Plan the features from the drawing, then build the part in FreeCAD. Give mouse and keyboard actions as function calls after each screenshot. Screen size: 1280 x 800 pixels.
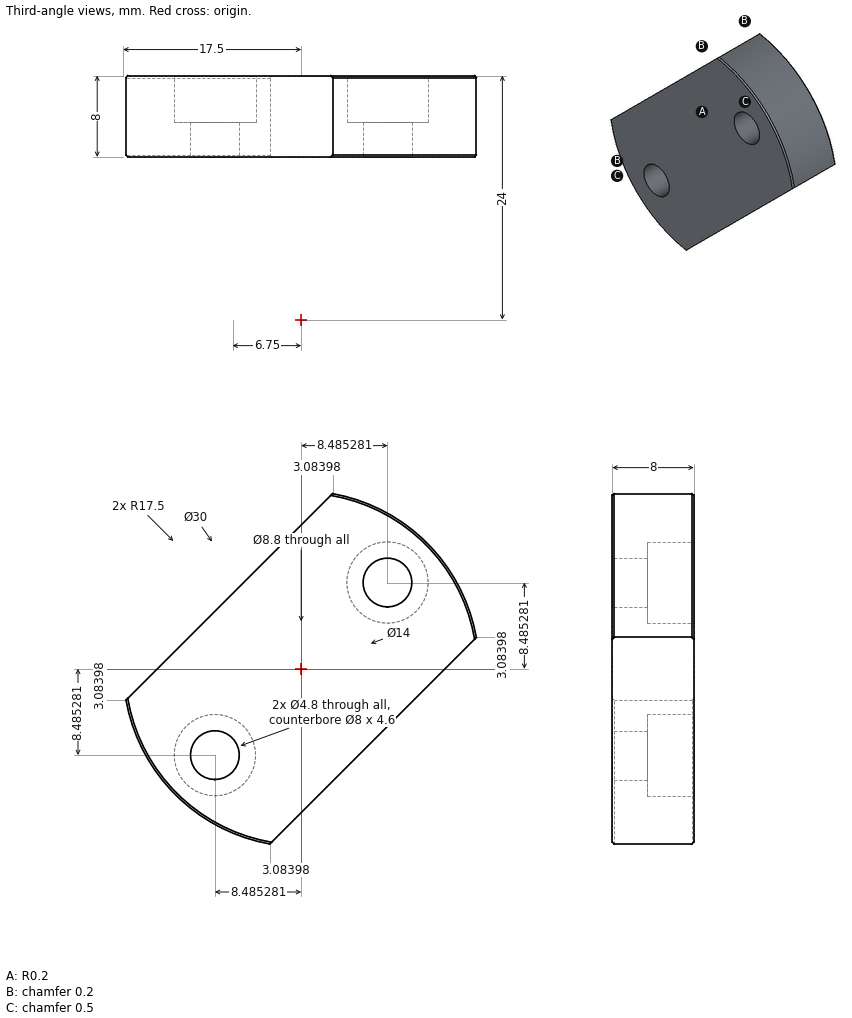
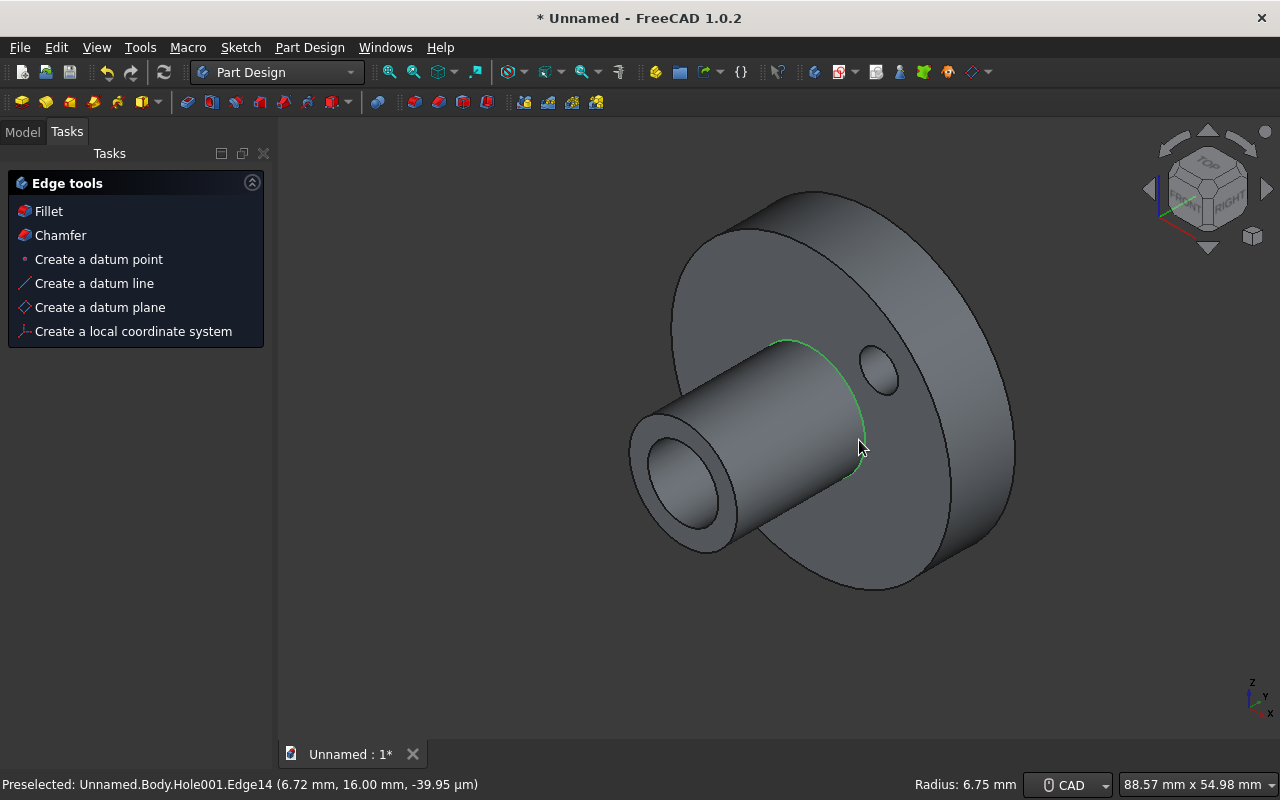
click(416, 102)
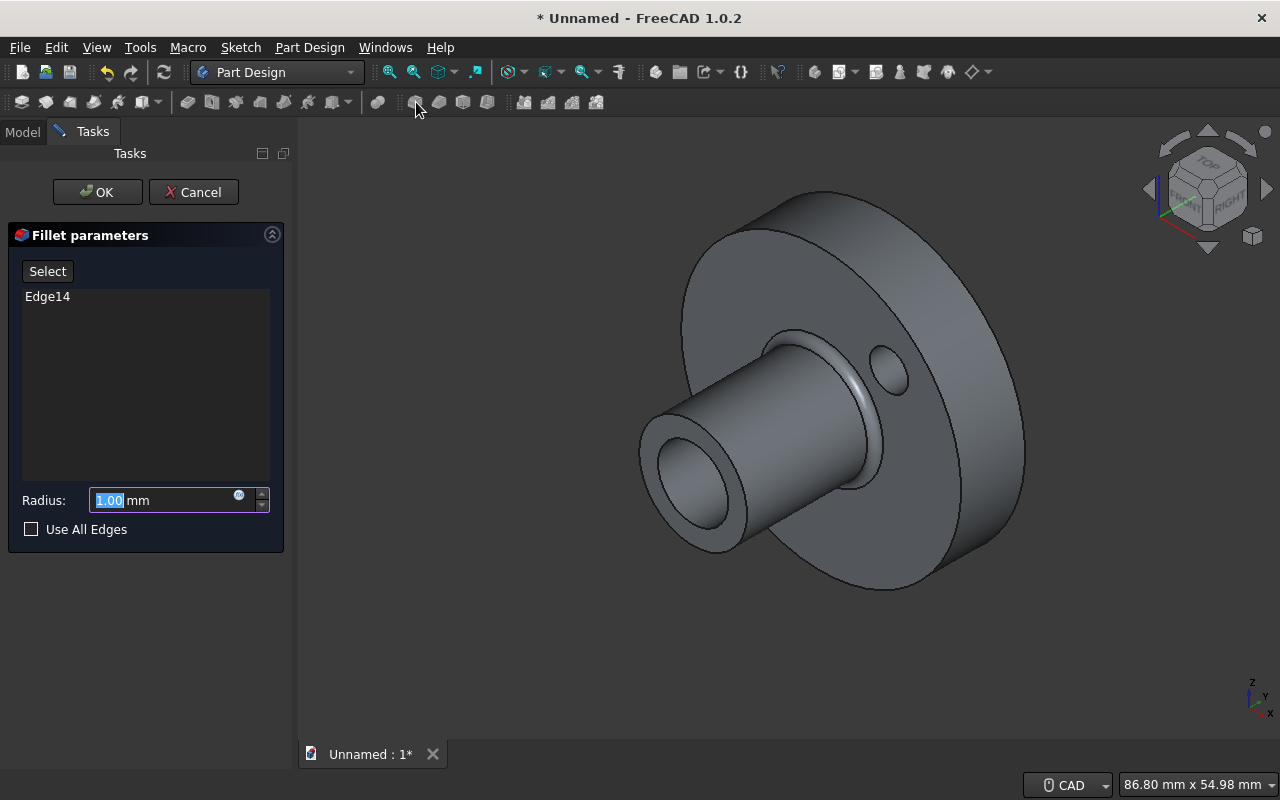
text(0.2)
key(Tab)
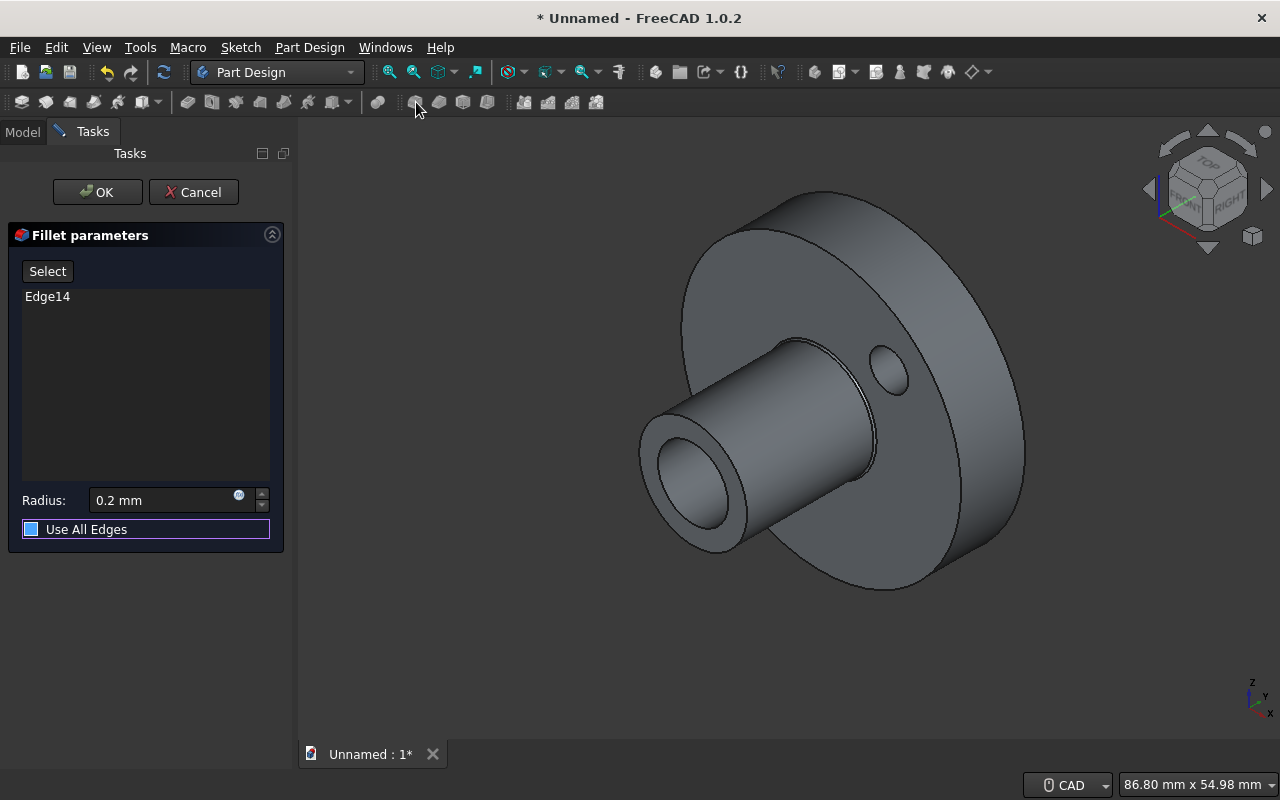
click(98, 192)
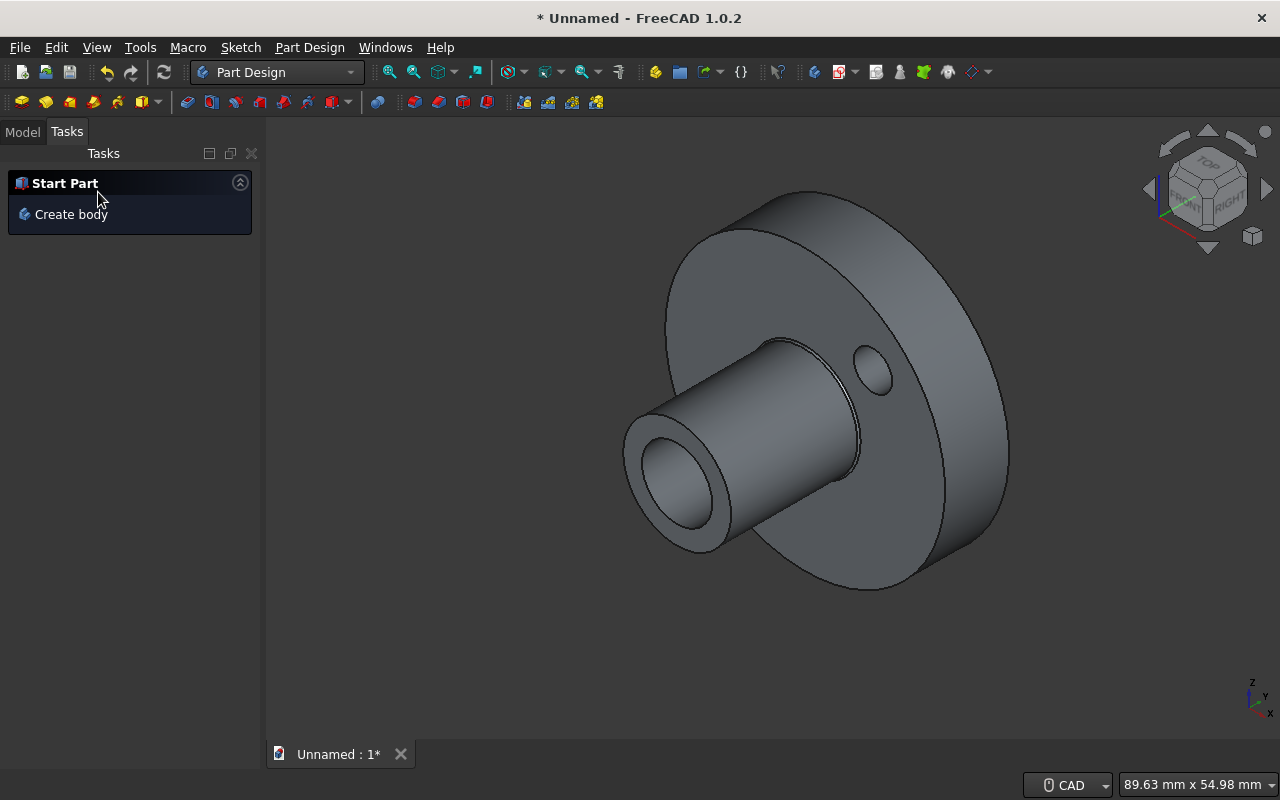
click(731, 514)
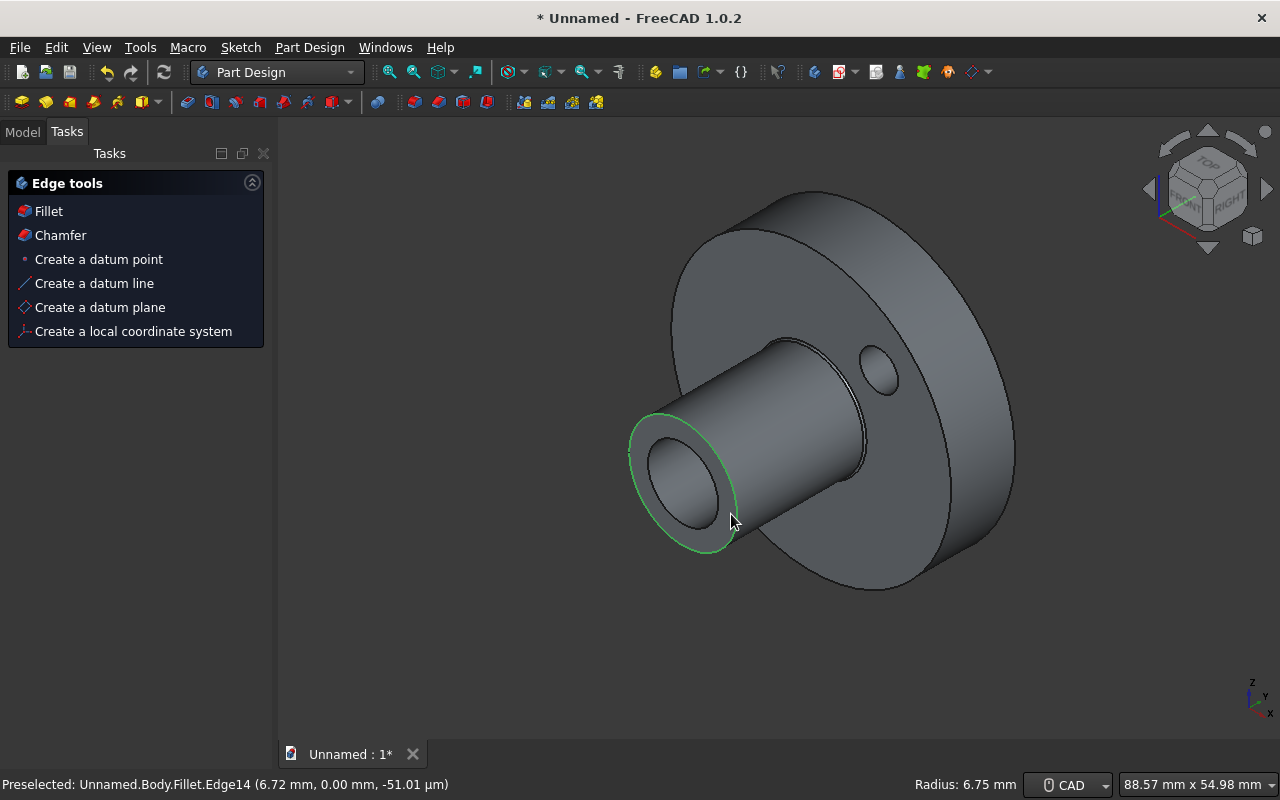
click(951, 489, ctrl)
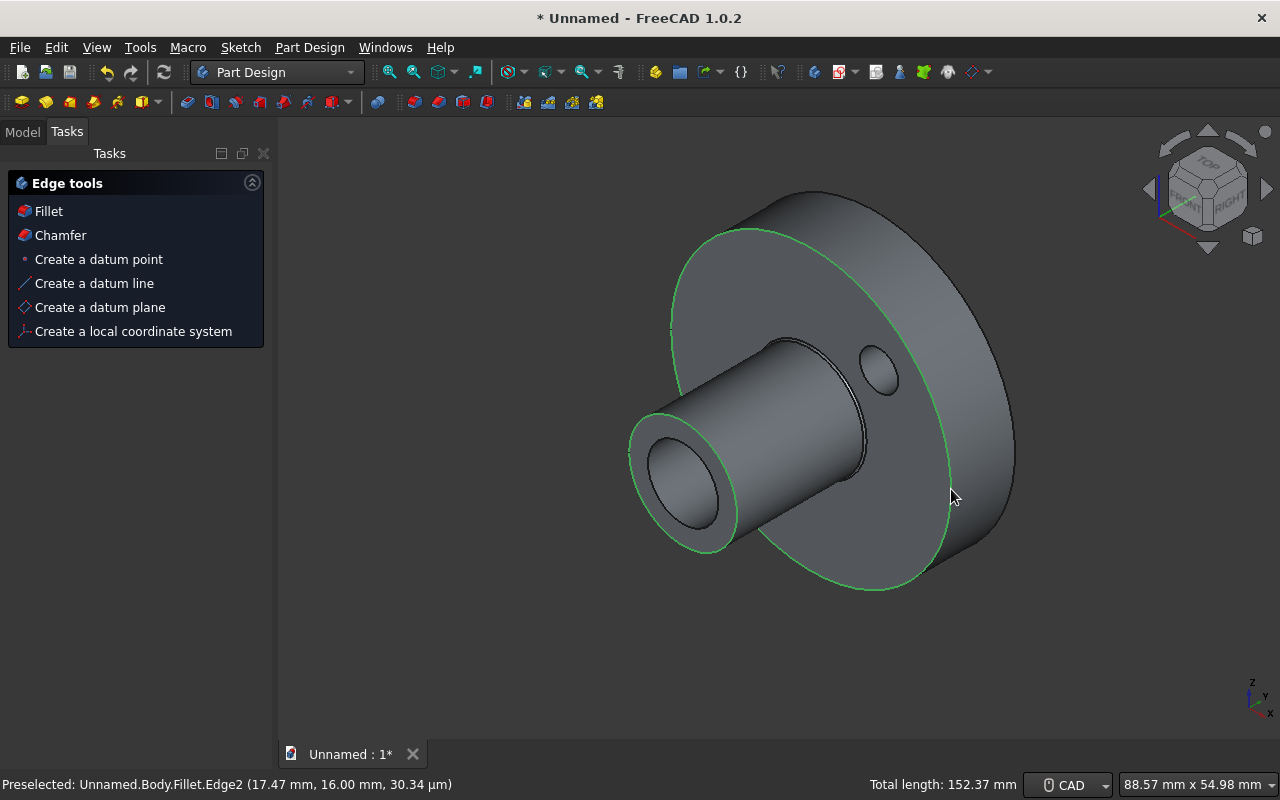
key(2)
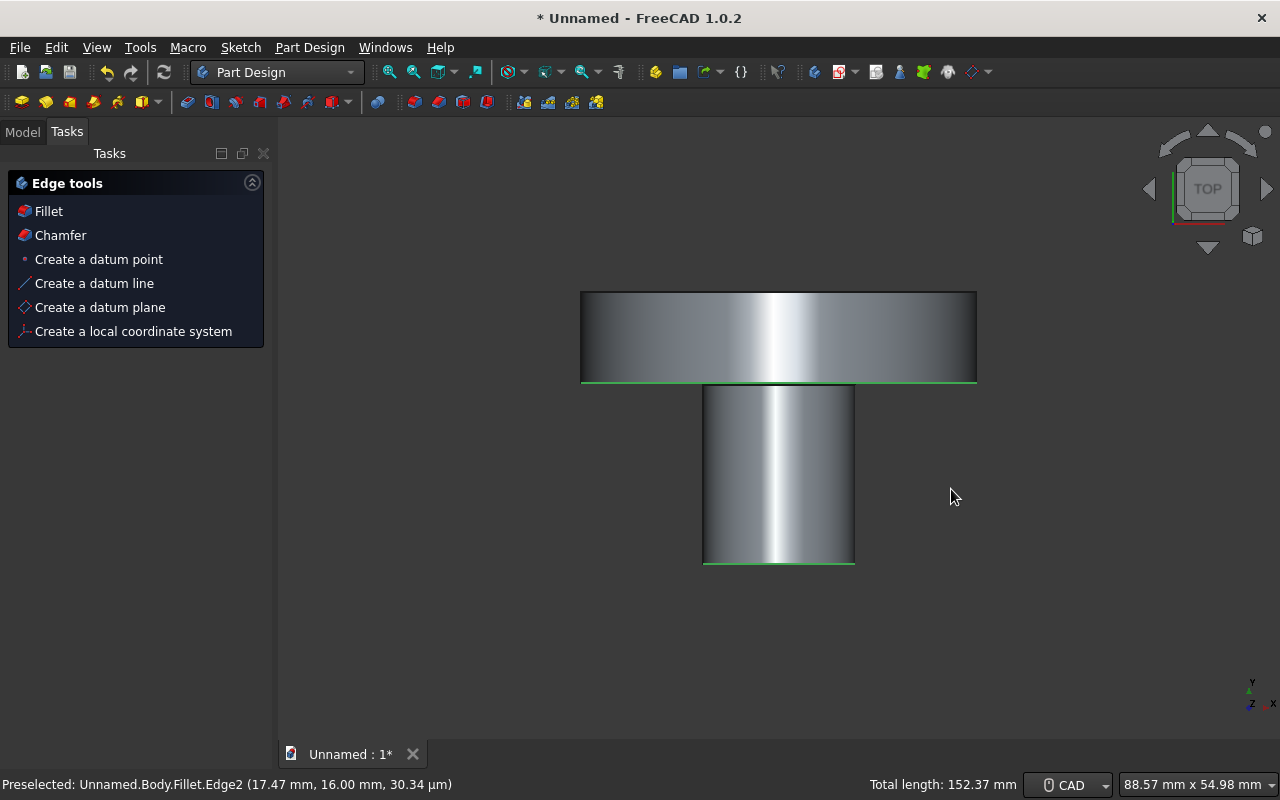
click(390, 72)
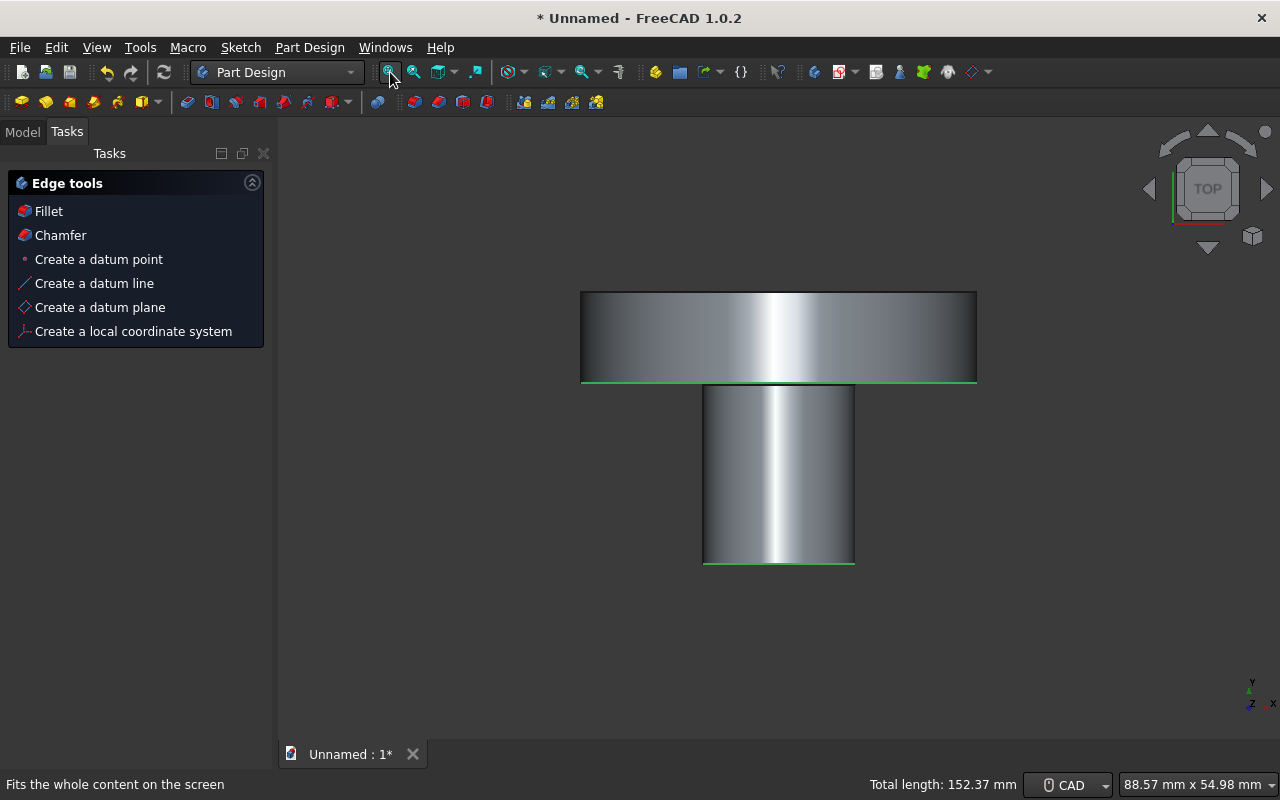
click(939, 291, ctrl)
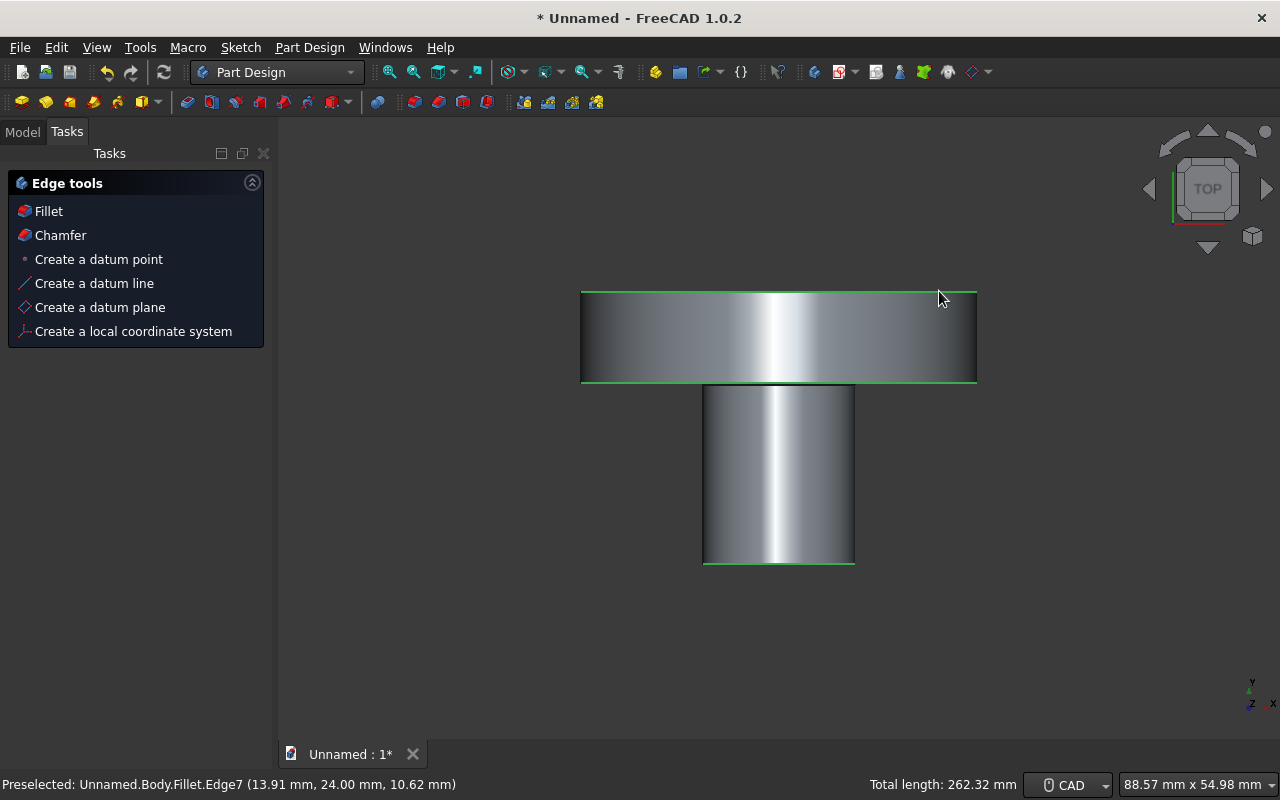
click(440, 102)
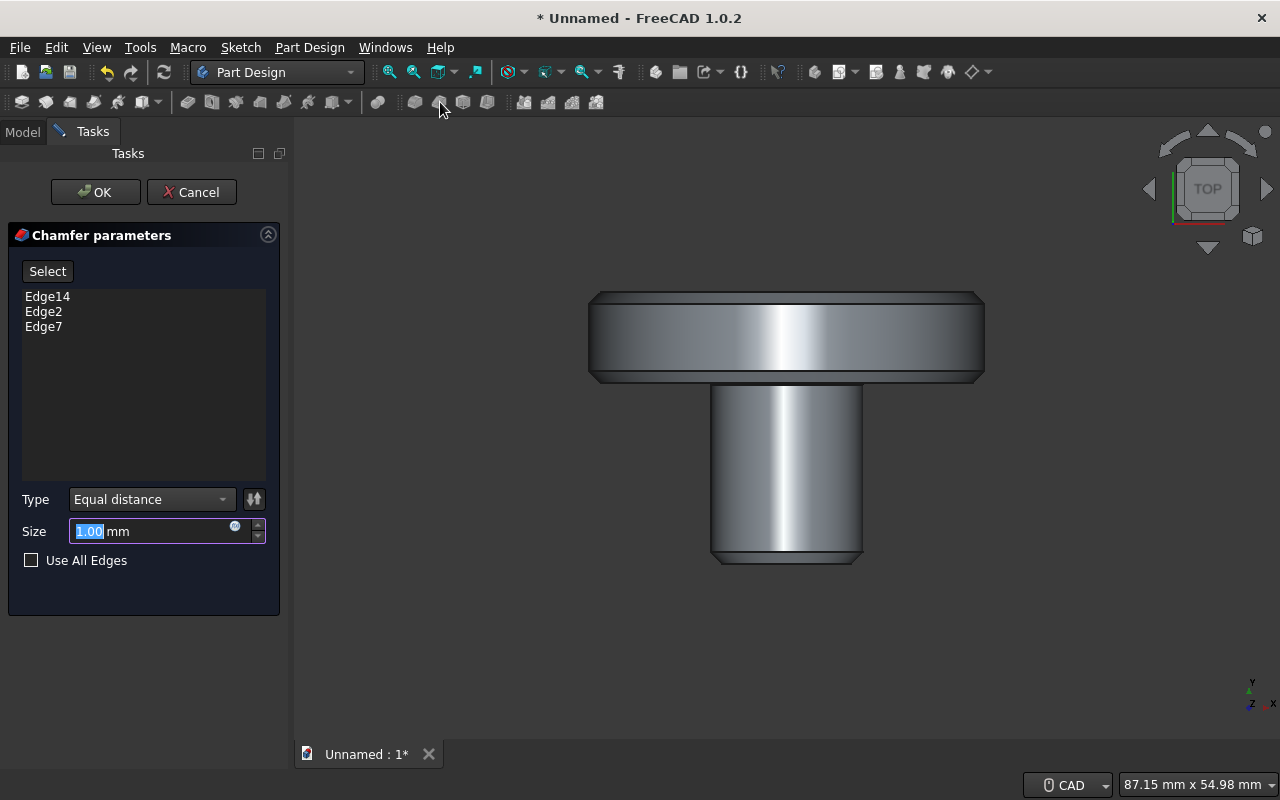
text(0.2)
key(Tab)